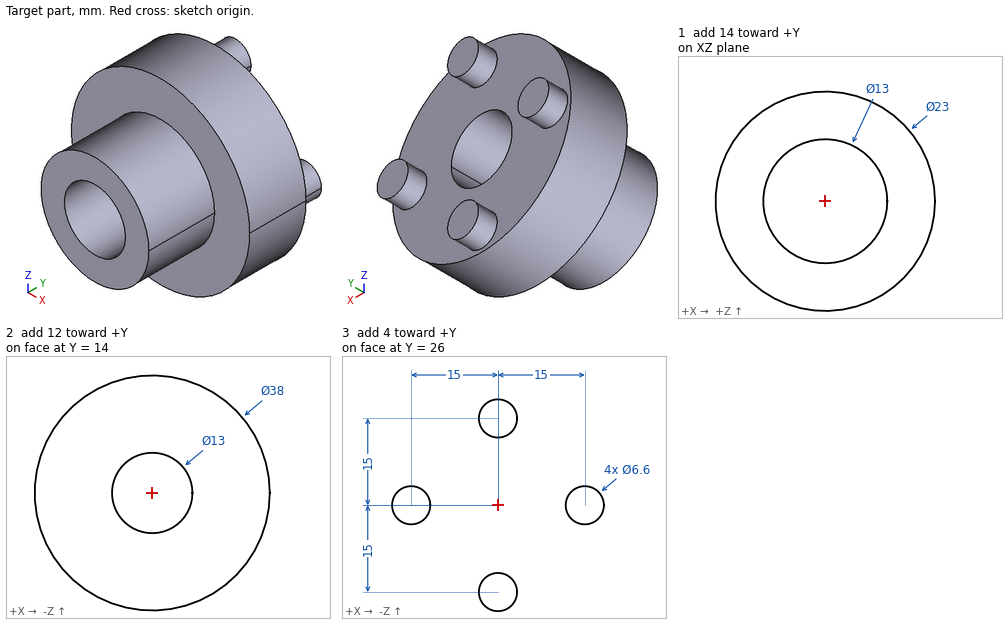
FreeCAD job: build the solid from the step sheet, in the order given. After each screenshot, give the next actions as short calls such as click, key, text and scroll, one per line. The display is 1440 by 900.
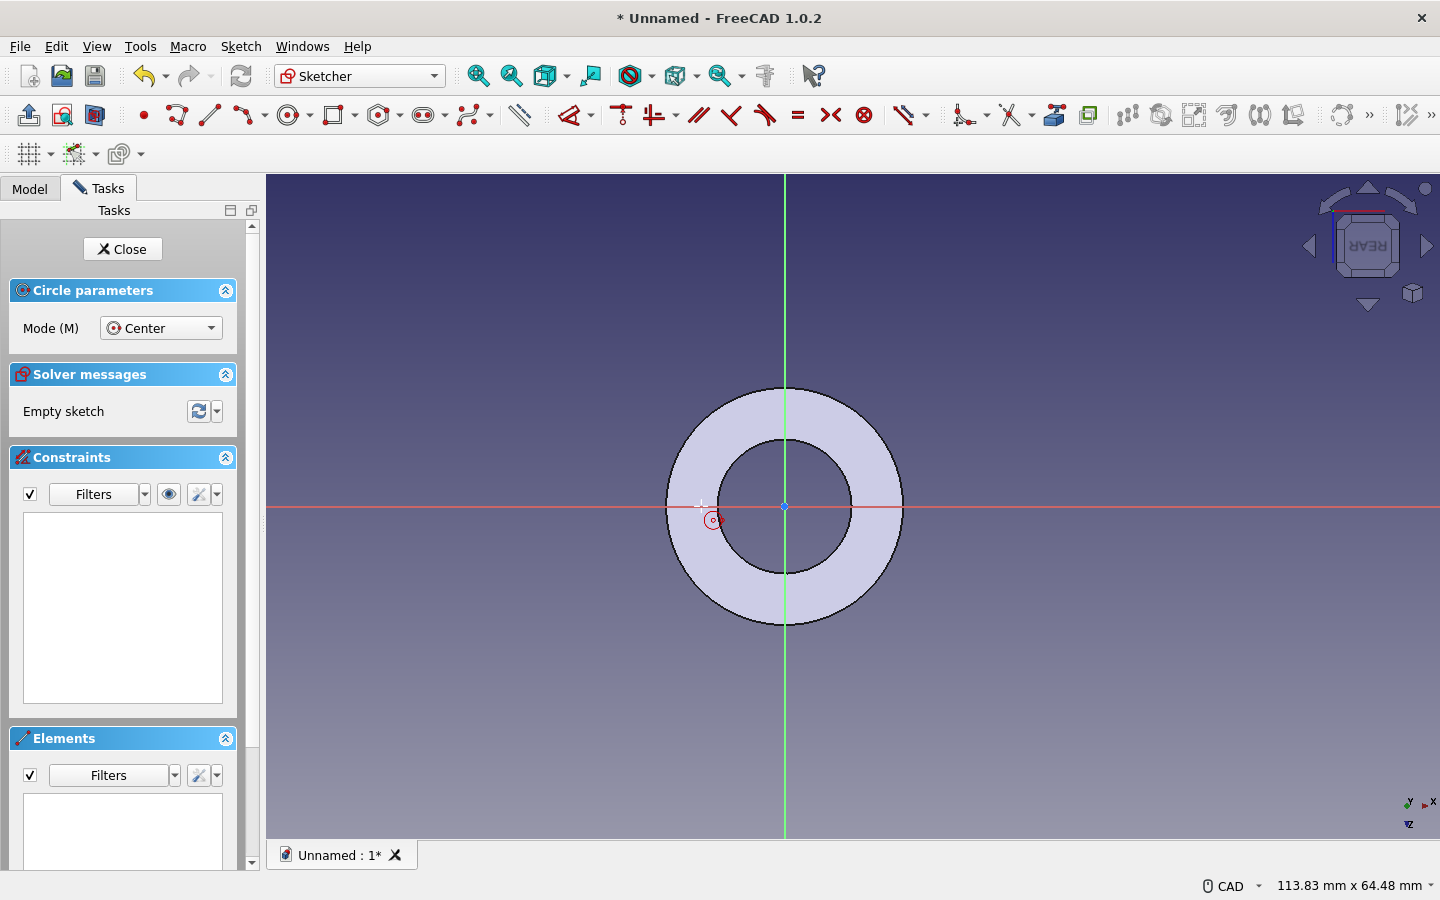
click(785, 507)
click(923, 368)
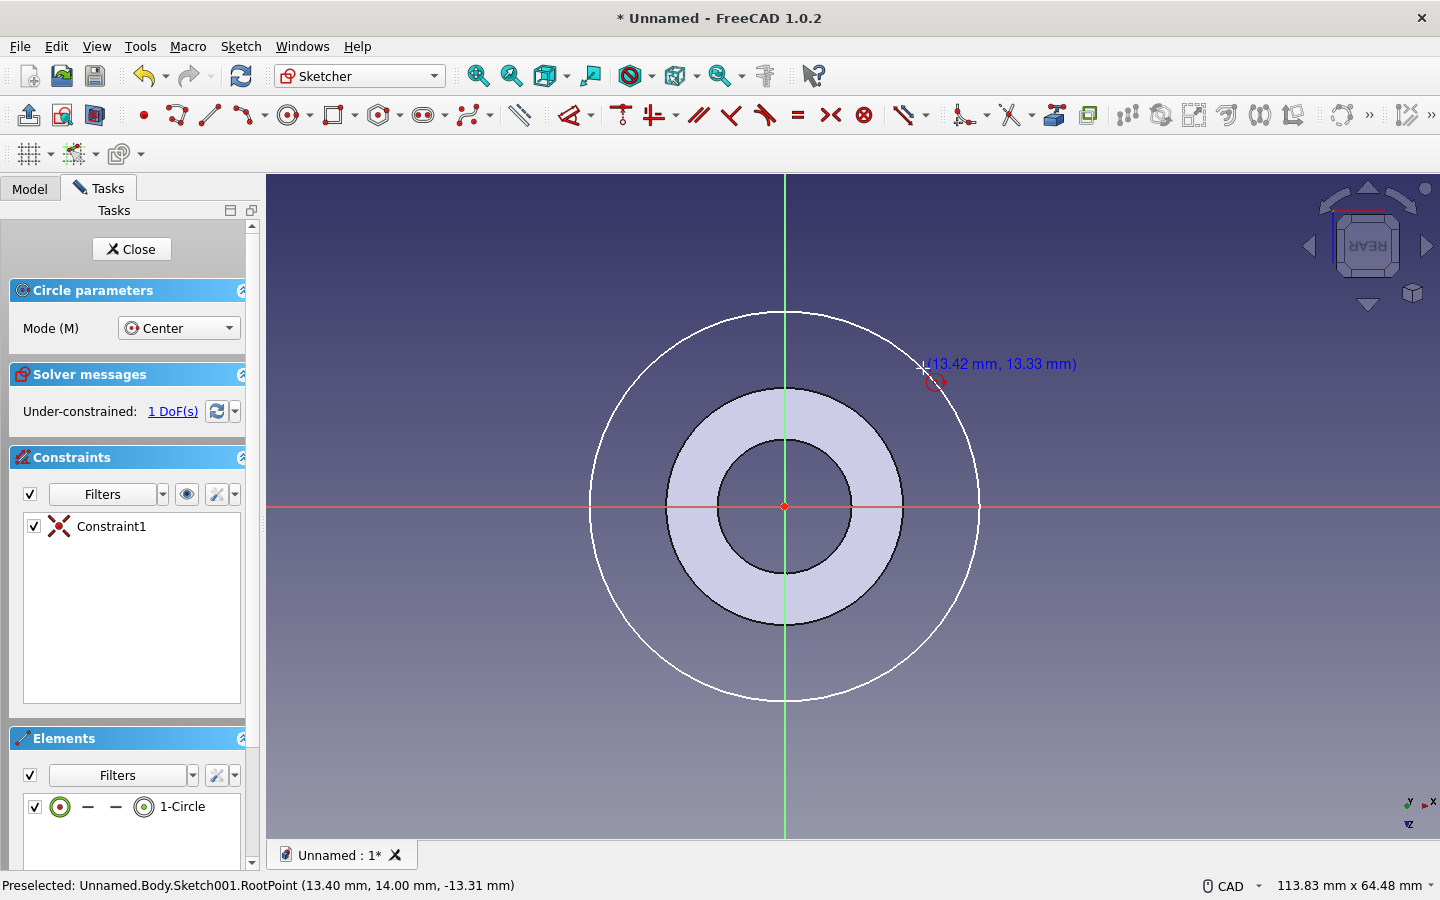
click(785, 507)
click(832, 459)
key(Escape)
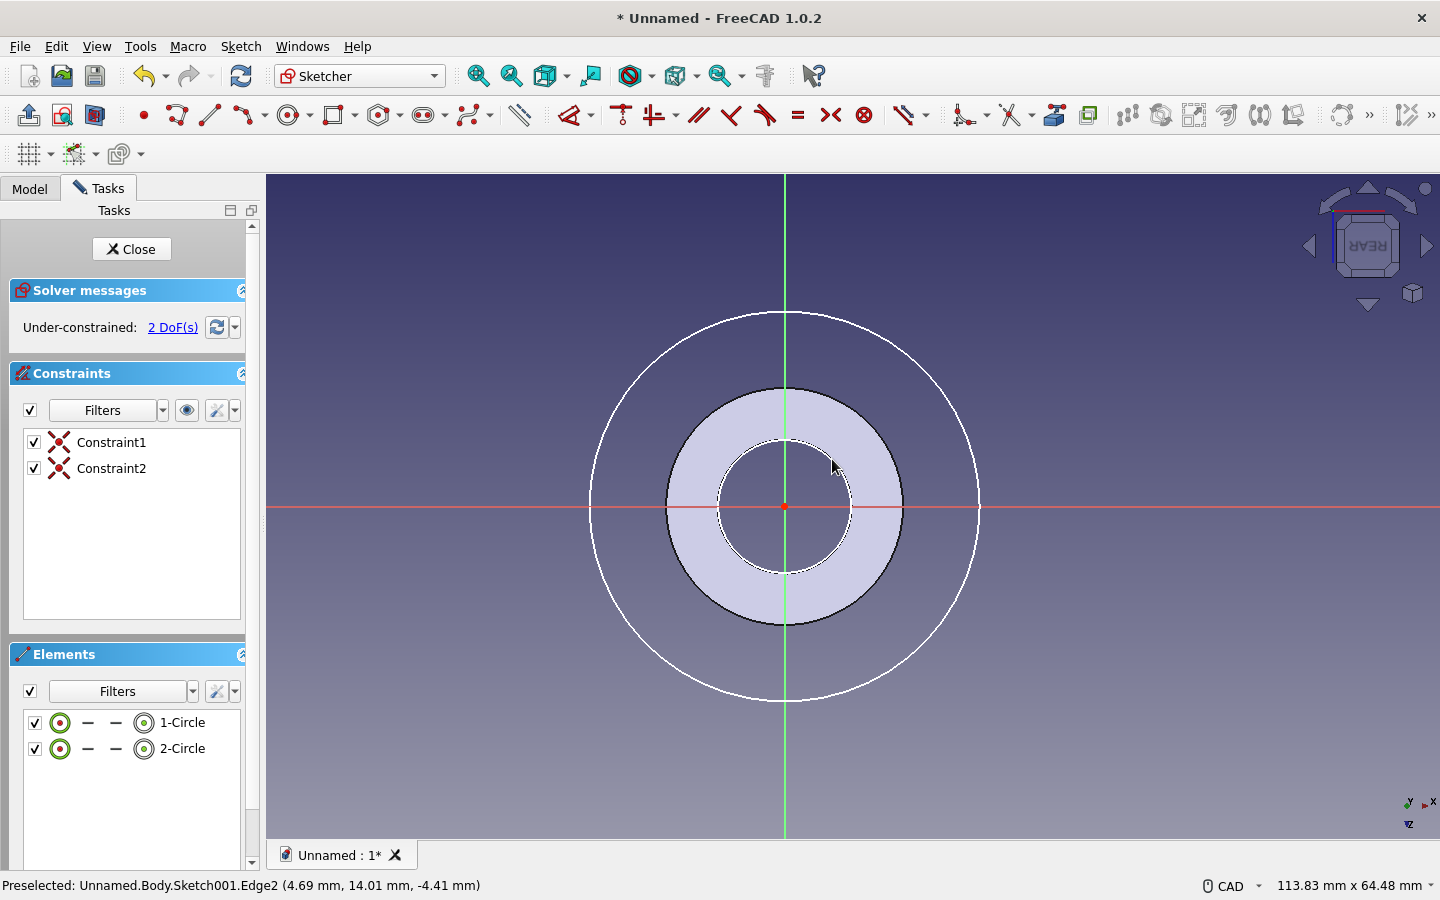
key(d)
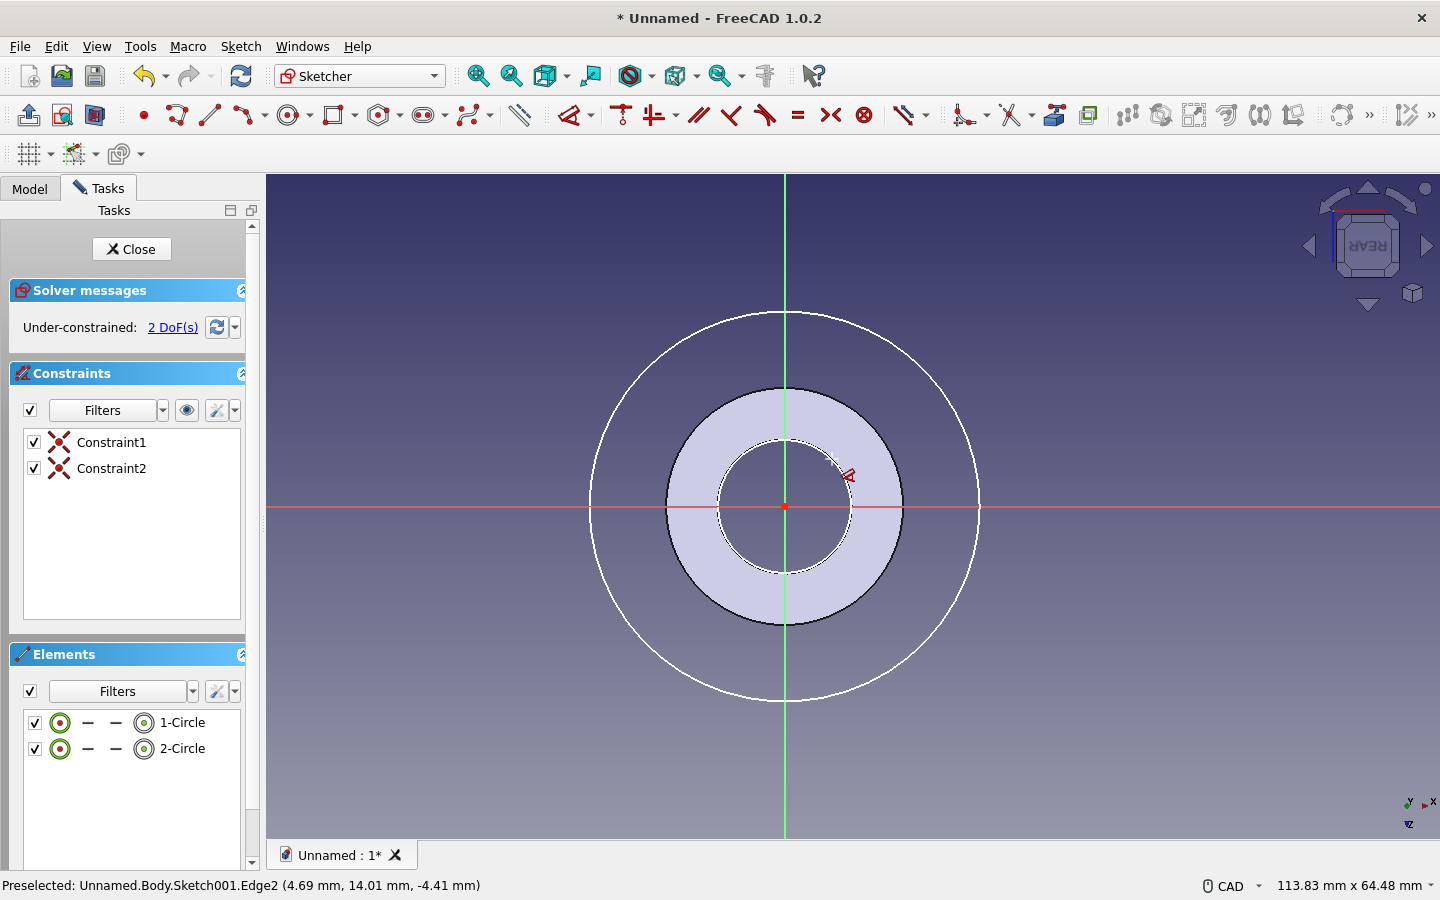
click(922, 368)
click(945, 345)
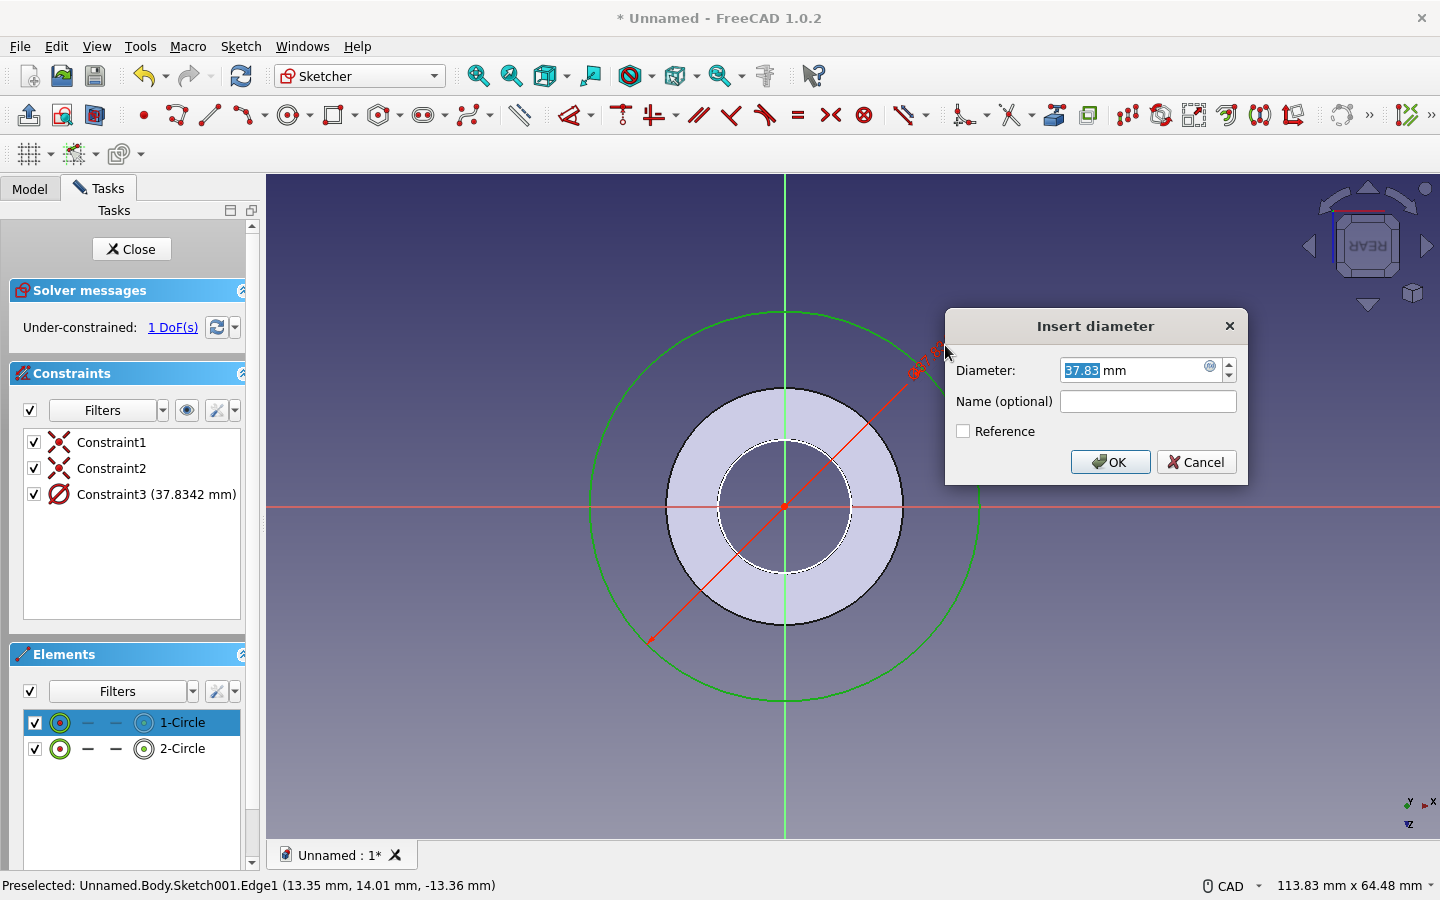
text(38)
key(Return)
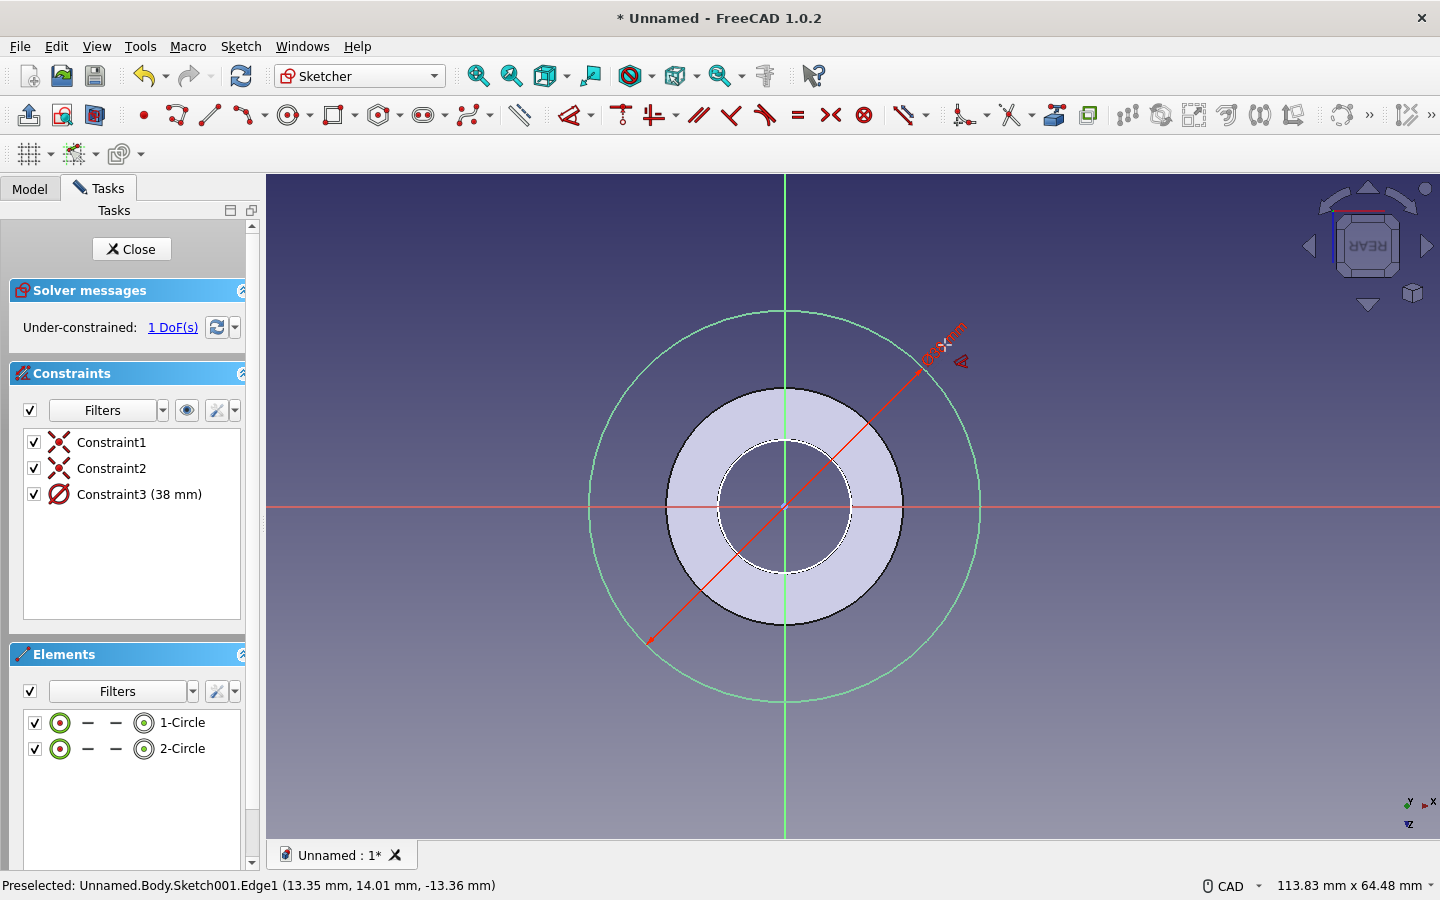
click(831, 459)
click(853, 436)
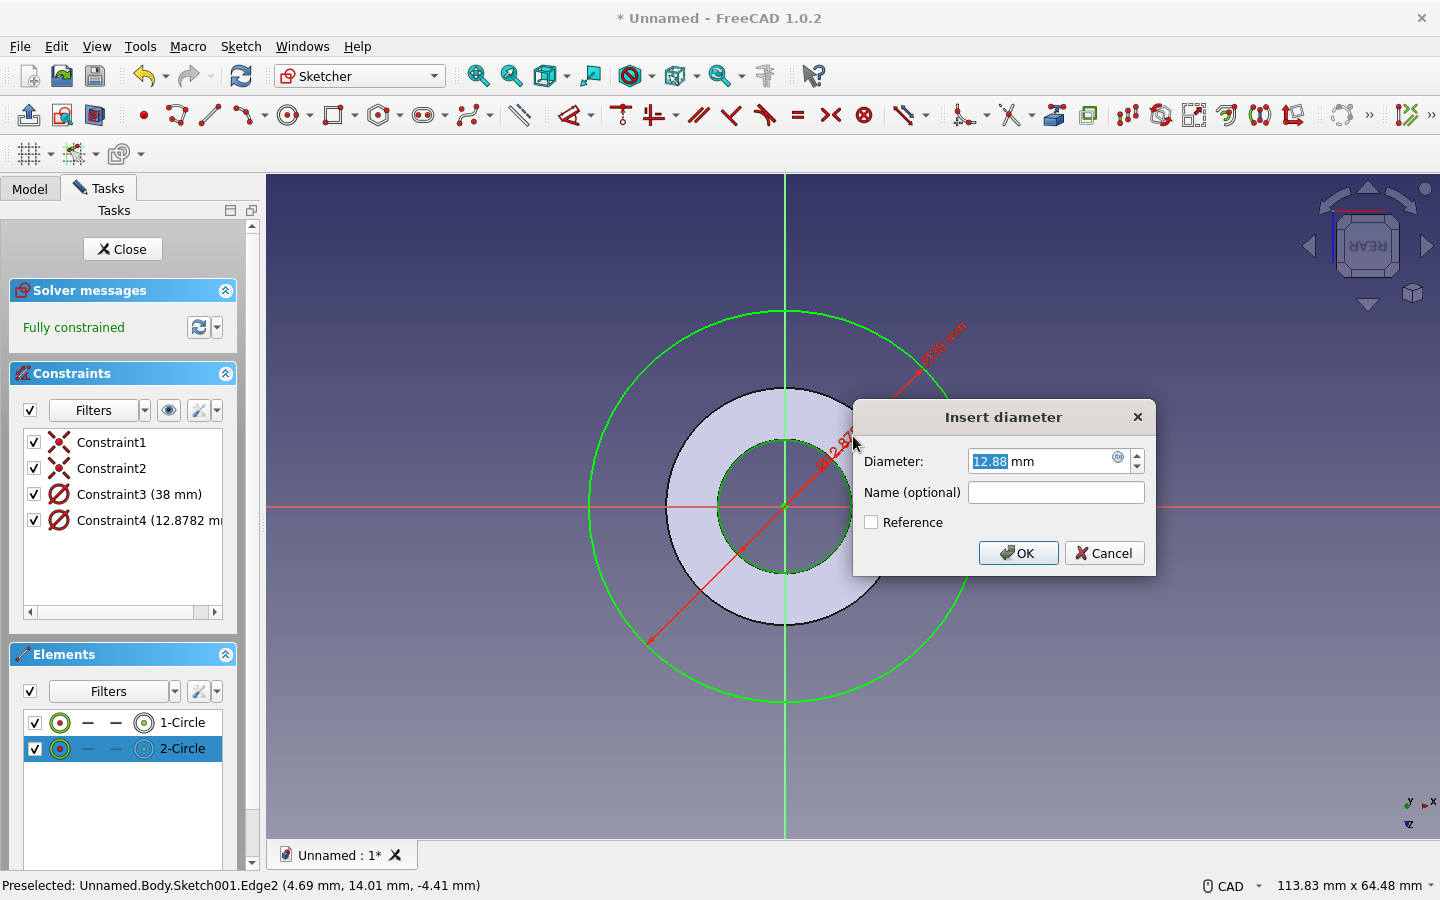
text(13)
key(Return)
key(Escape)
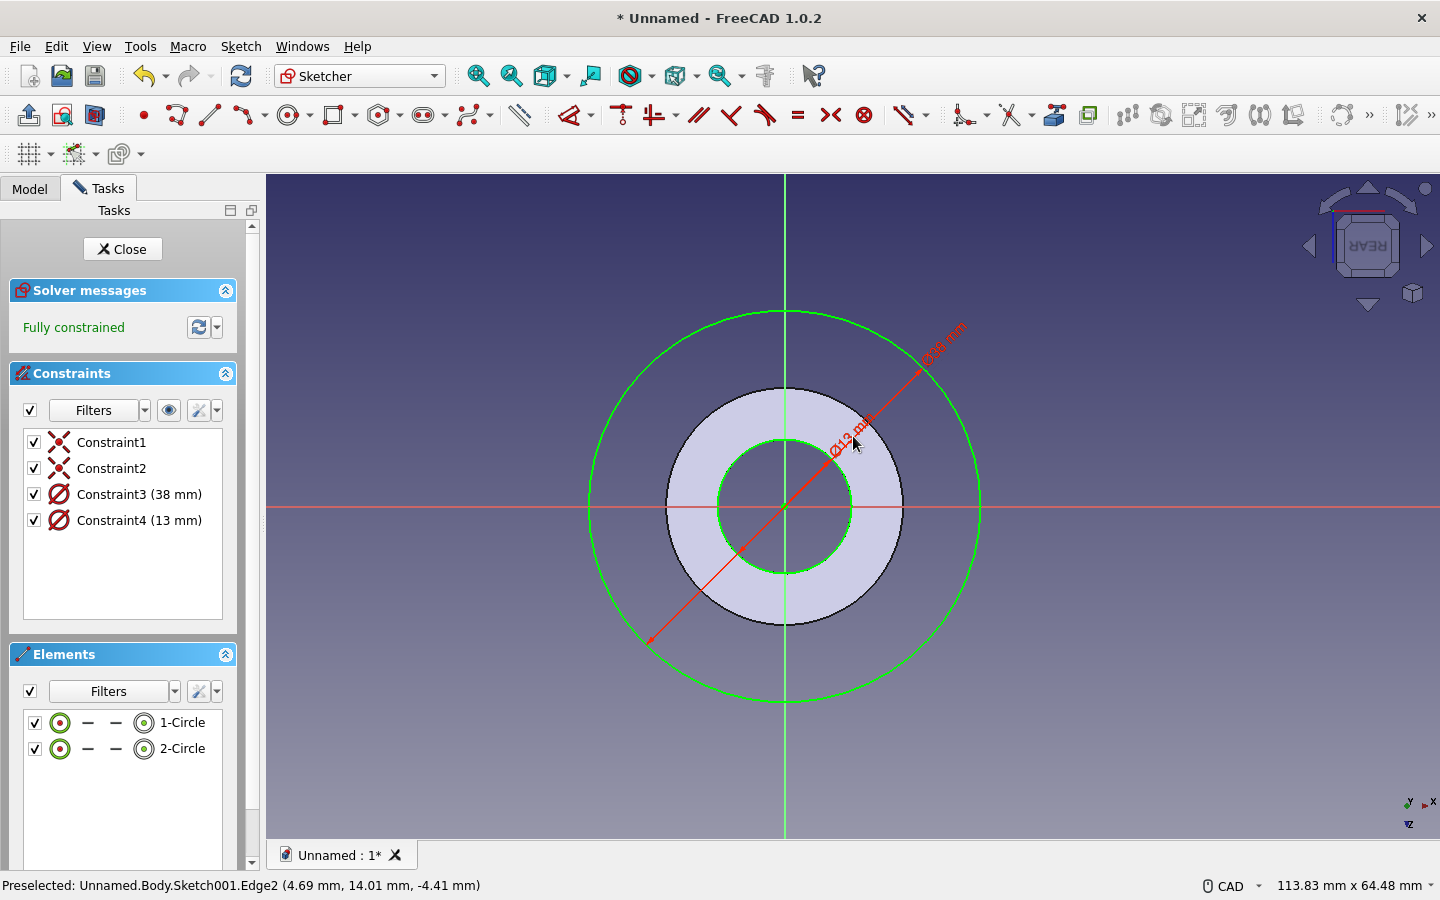
click(123, 249)